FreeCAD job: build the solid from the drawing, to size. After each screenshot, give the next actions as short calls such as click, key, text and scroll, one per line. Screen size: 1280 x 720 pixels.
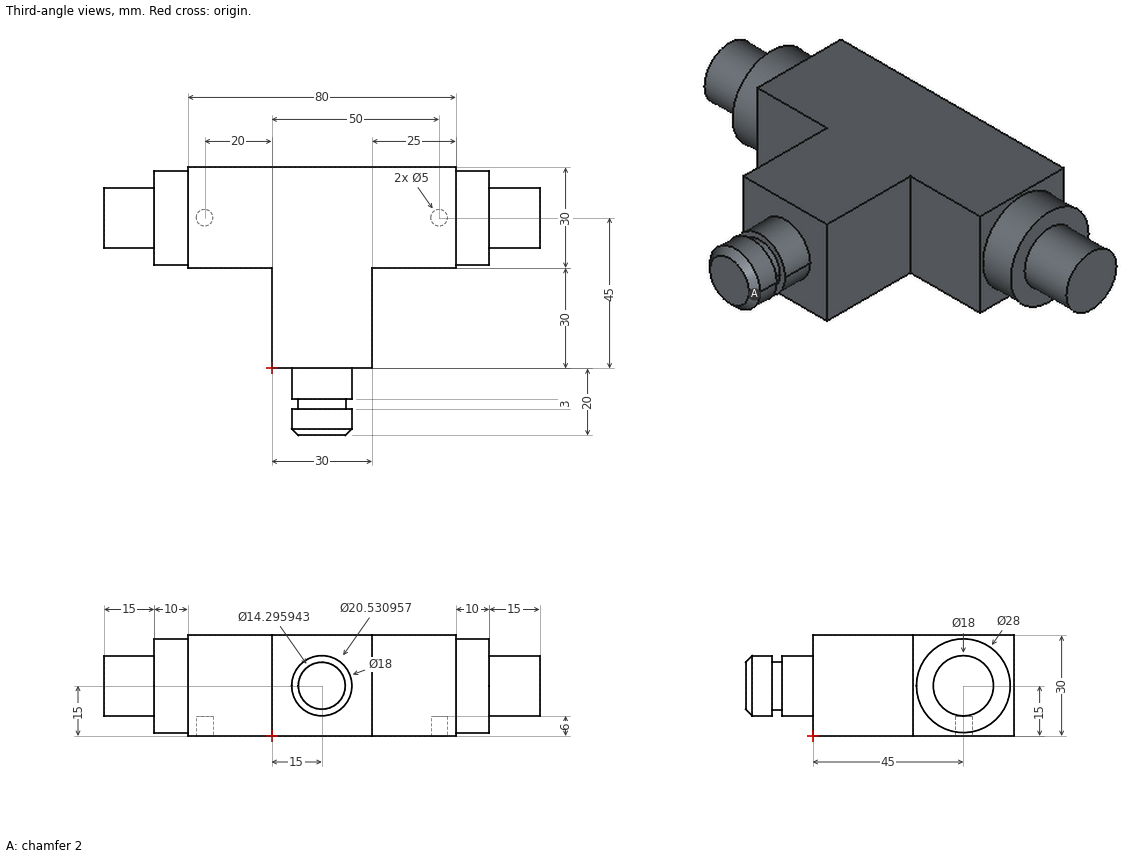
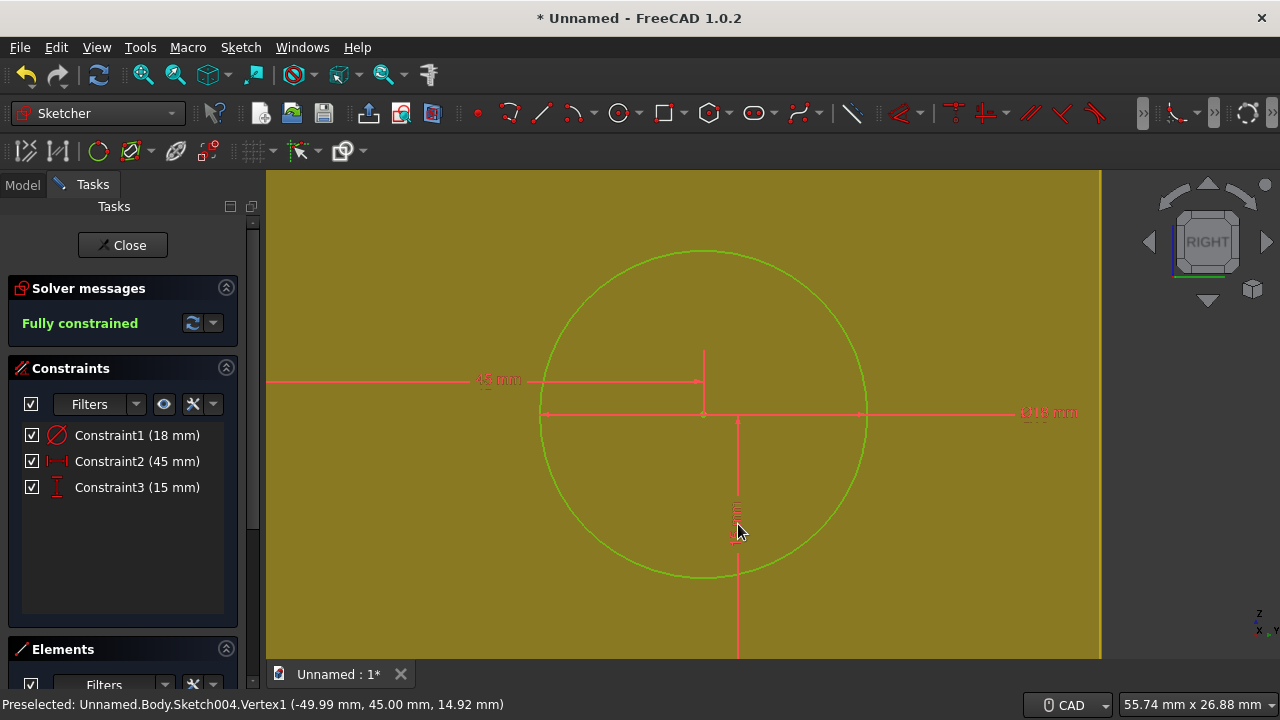
click(123, 245)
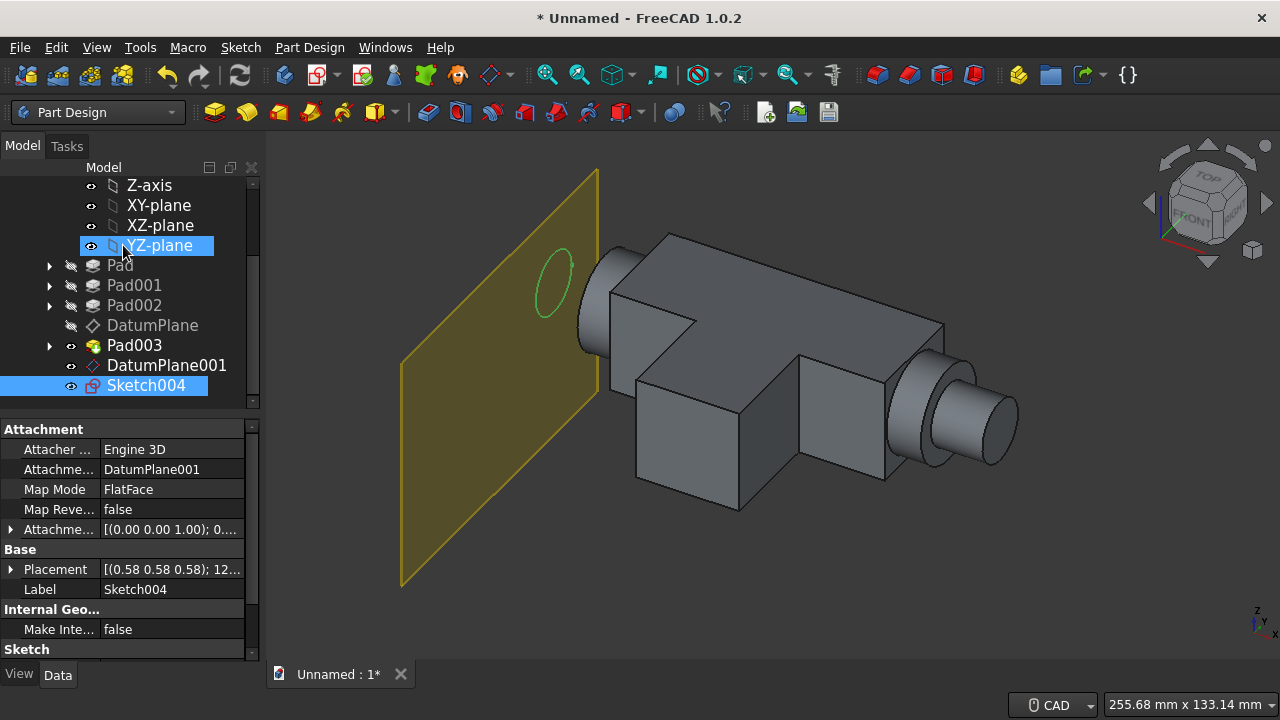
click(216, 112)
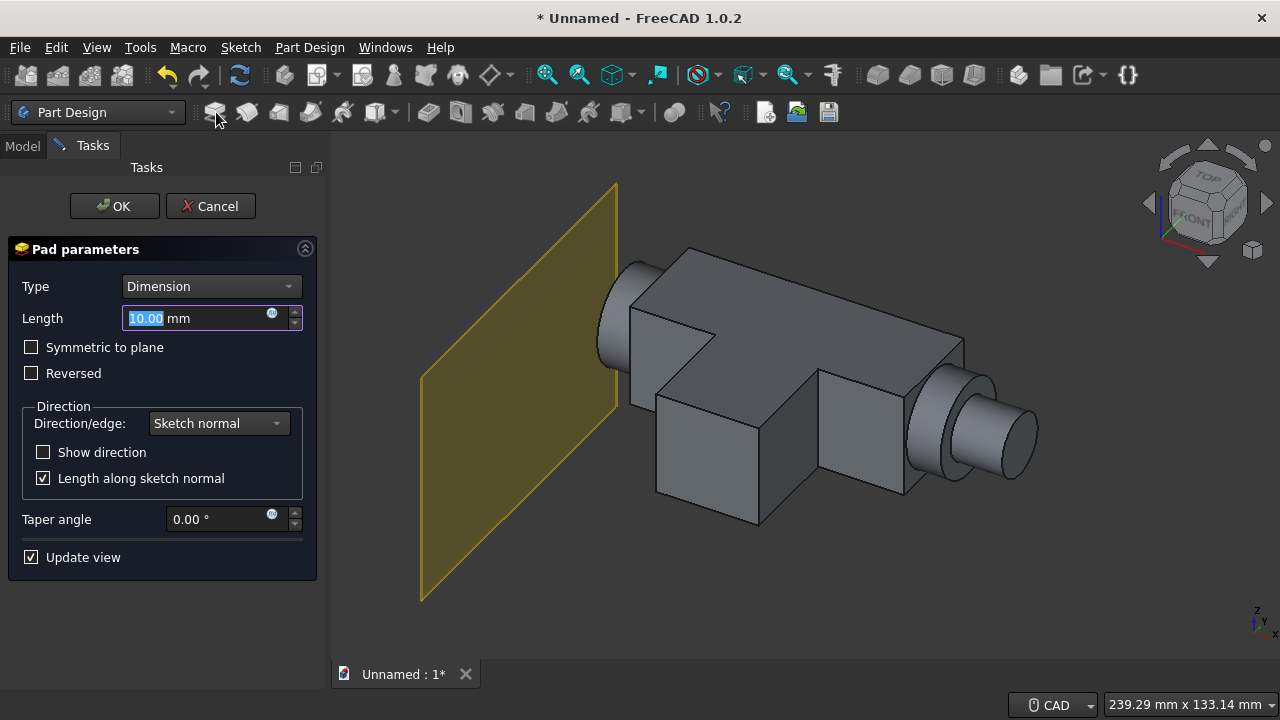
text(15)
key(Tab)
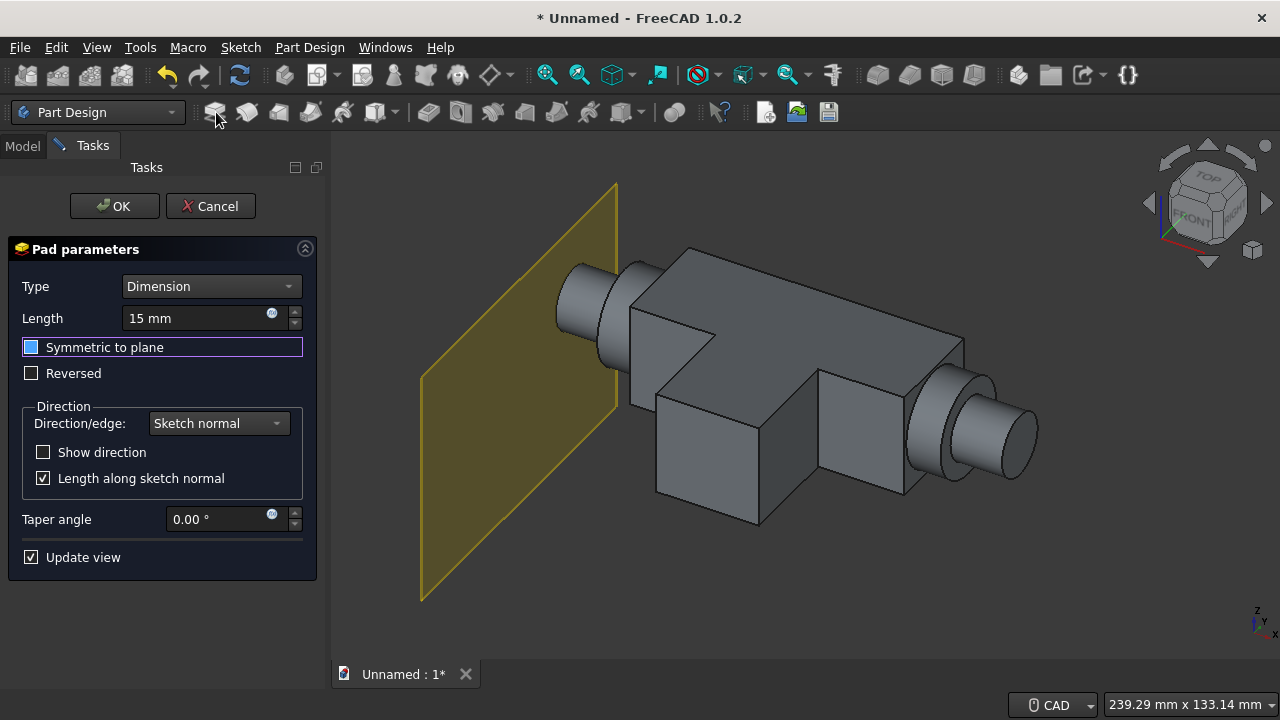
click(115, 206)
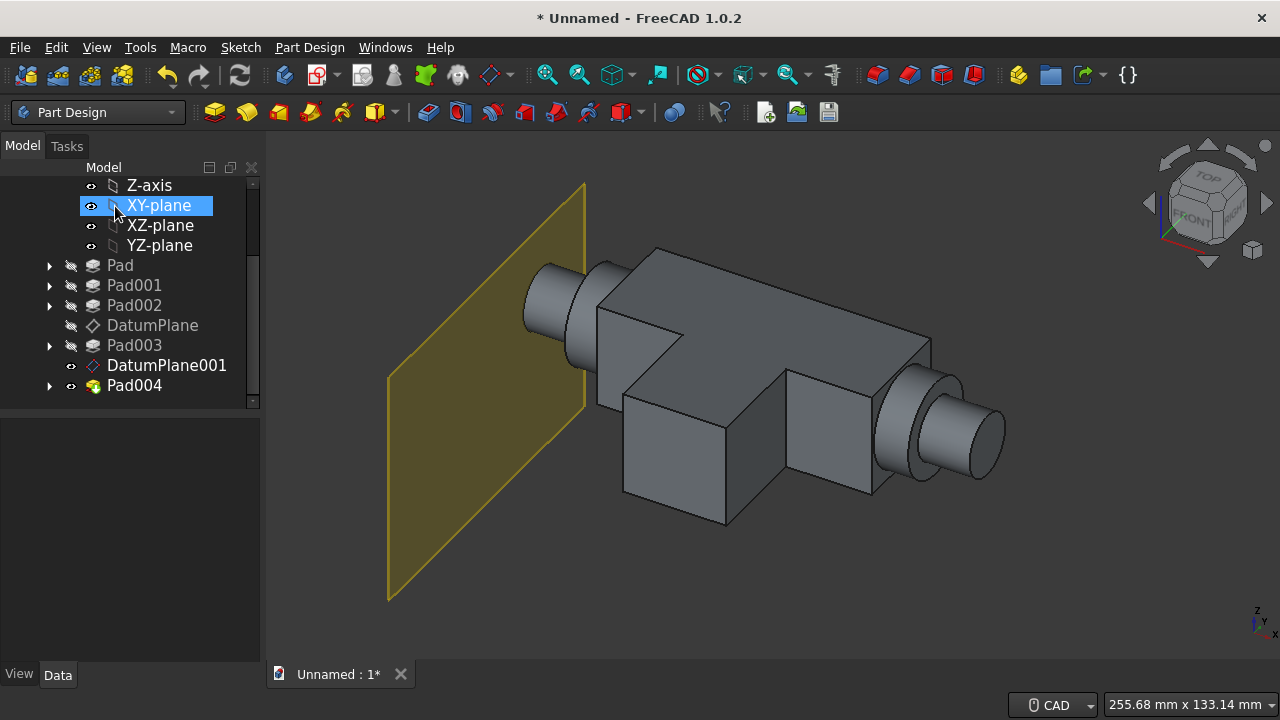
click(116, 366)
key(space)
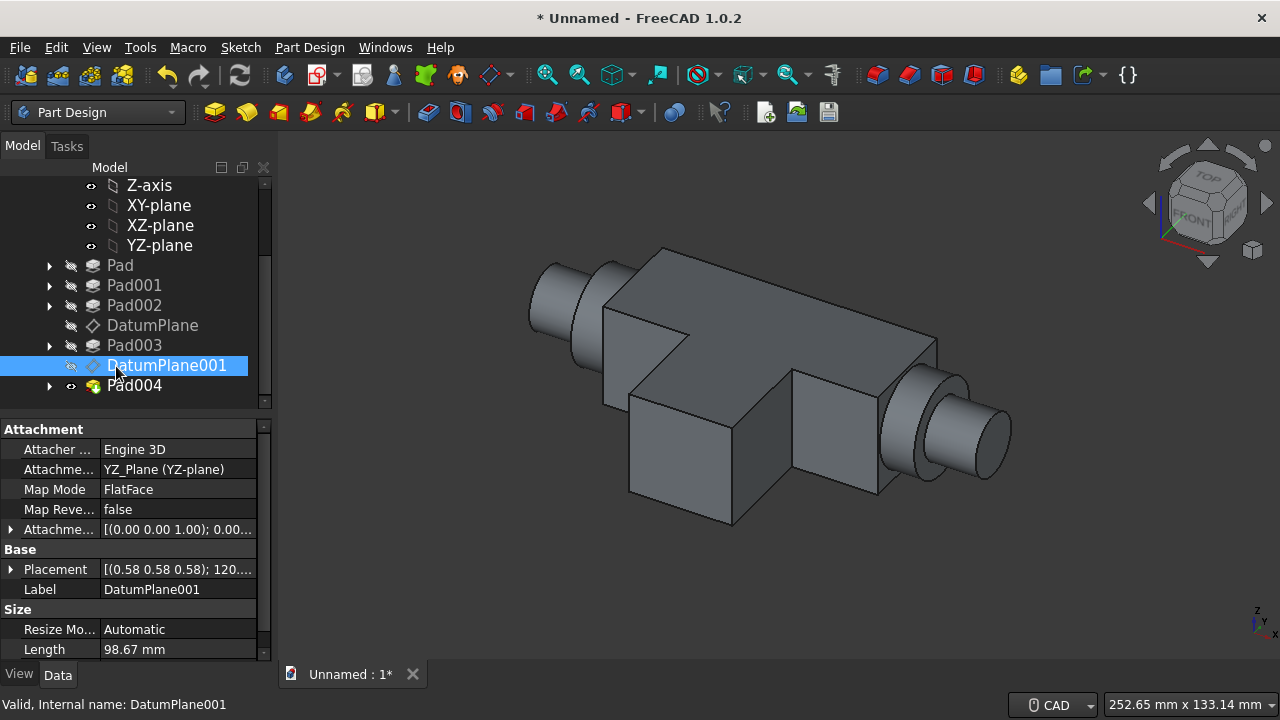
click(681, 459)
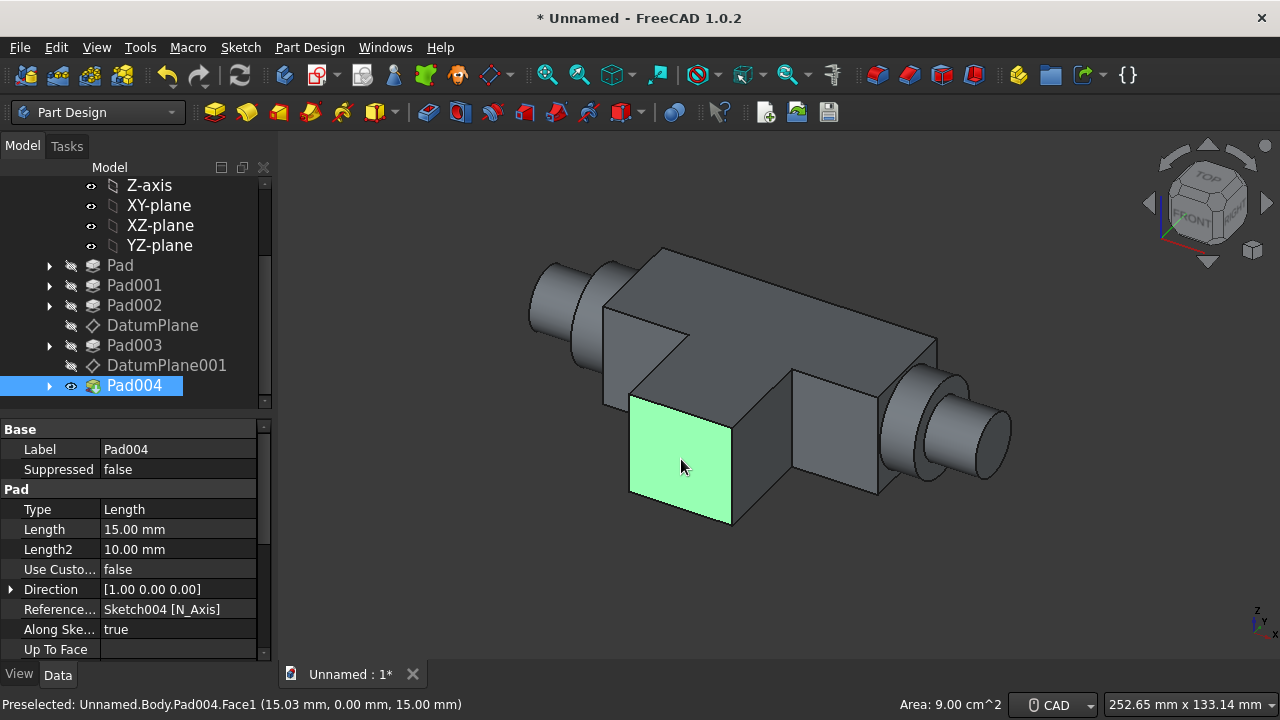
click(318, 76)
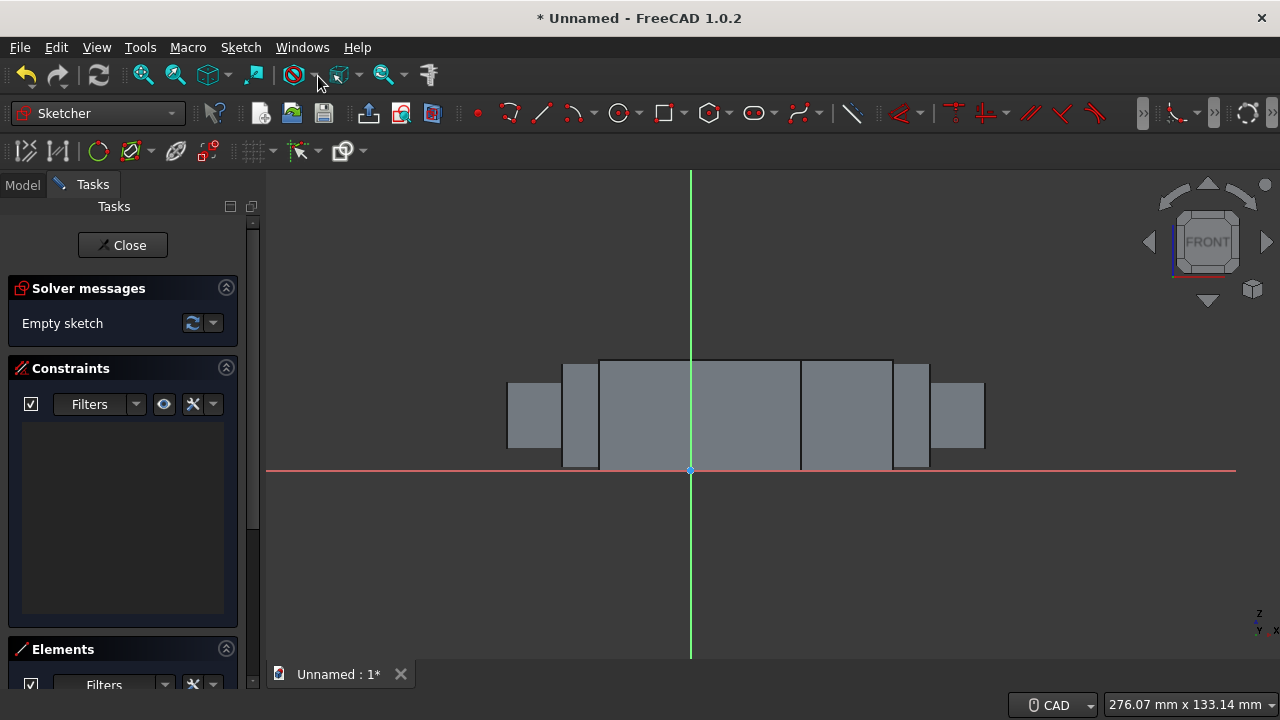
scroll(748, 432, up, 6)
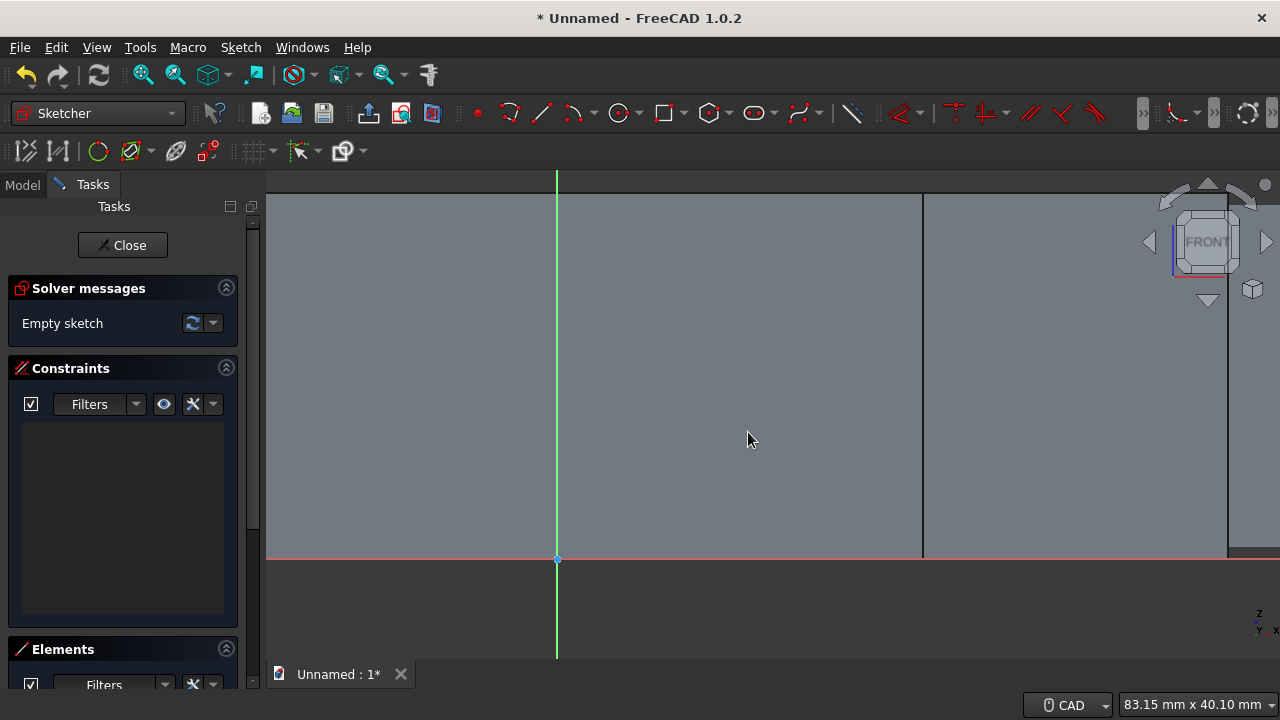
key(g)
key(c)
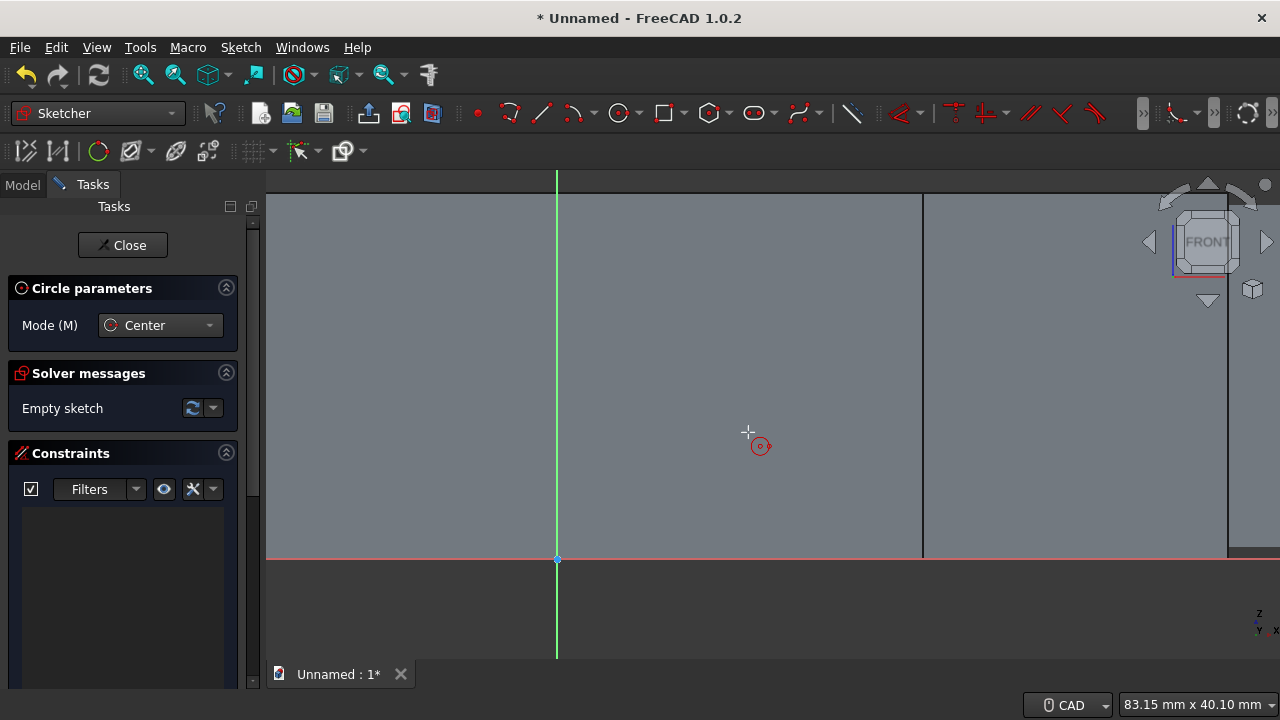
click(740, 376)
move(818, 299)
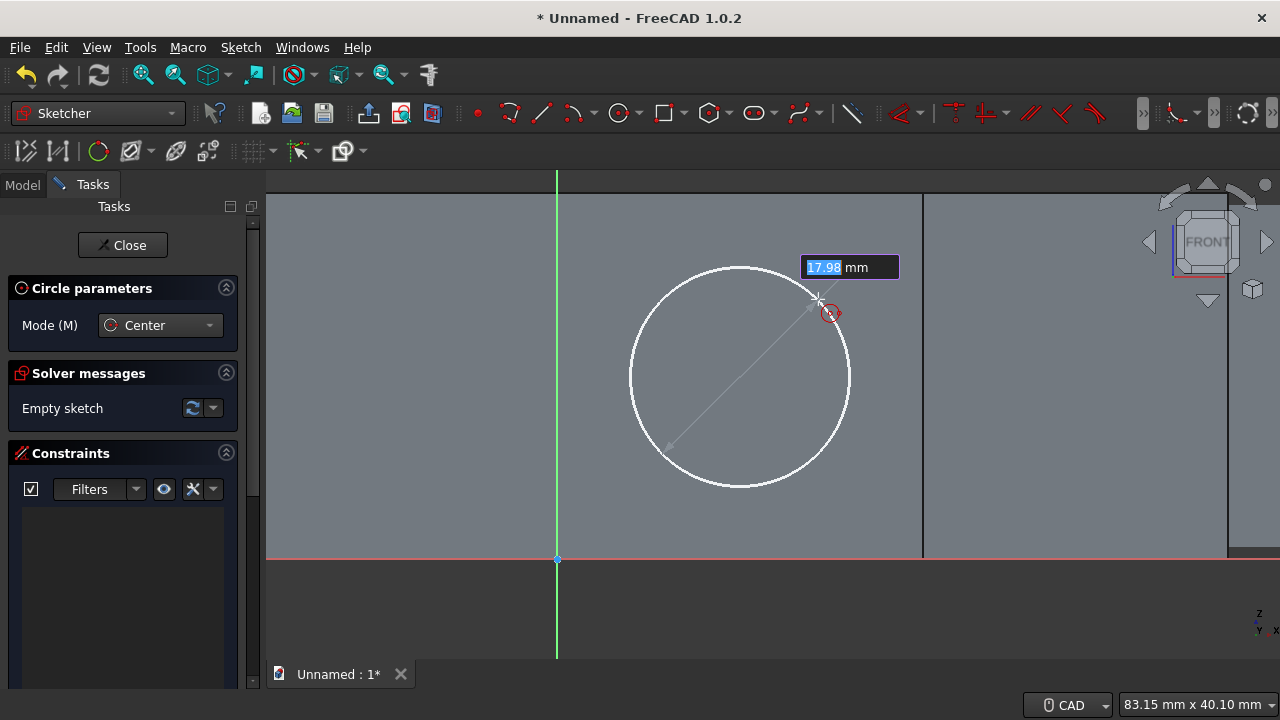
text(18)
key(Return)
key(Escape)